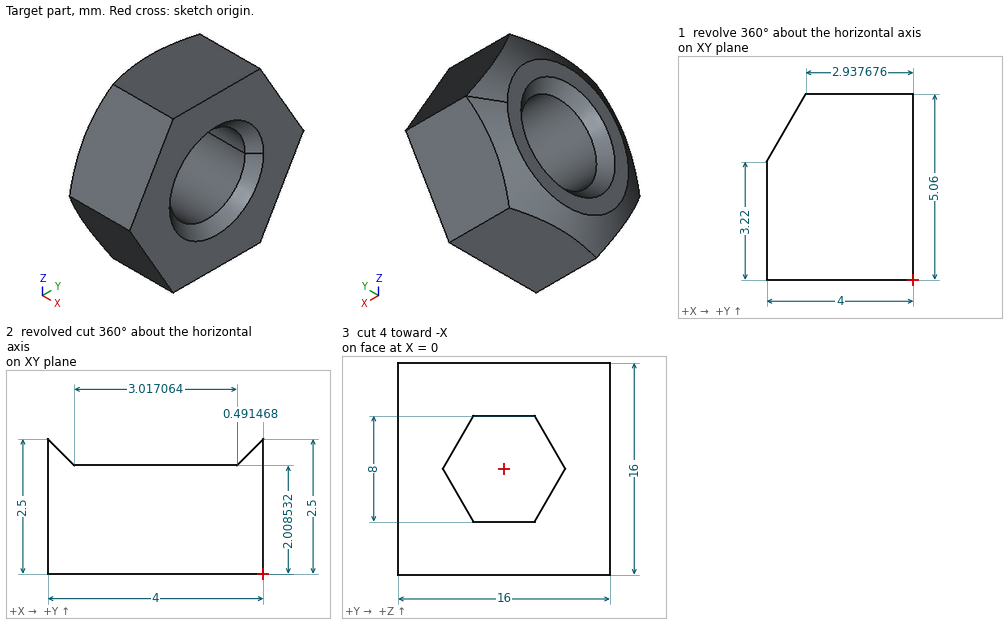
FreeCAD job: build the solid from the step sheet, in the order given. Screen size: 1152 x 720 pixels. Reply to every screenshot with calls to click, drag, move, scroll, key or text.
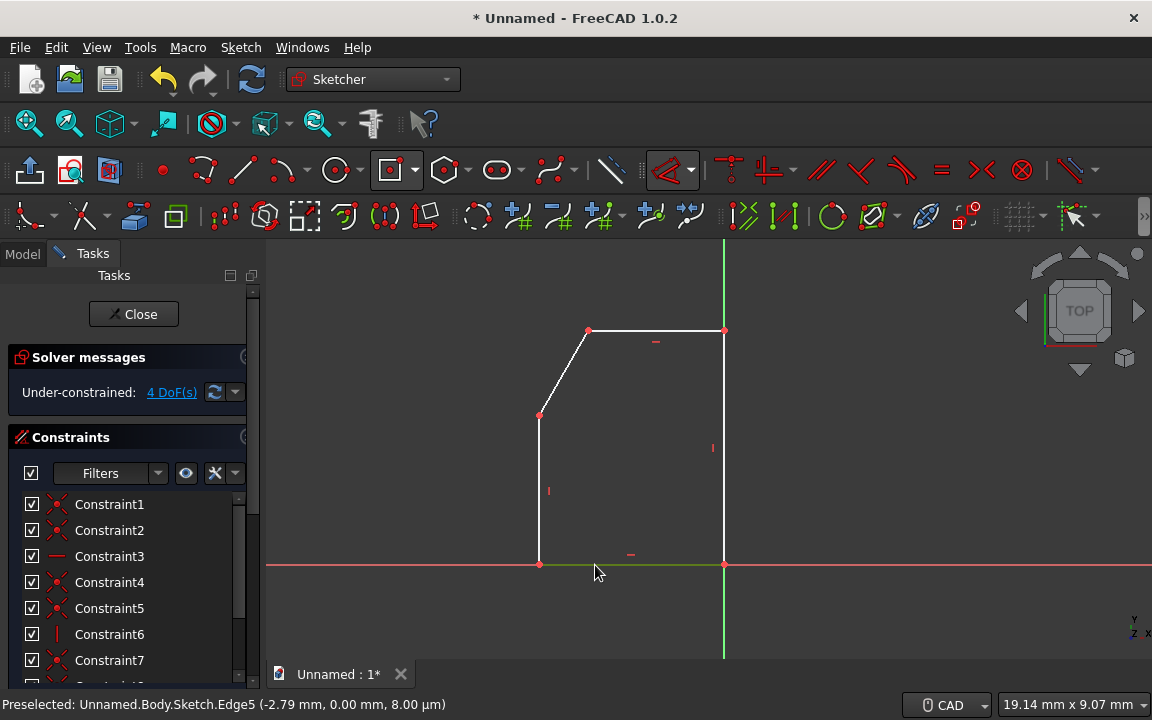
key(l)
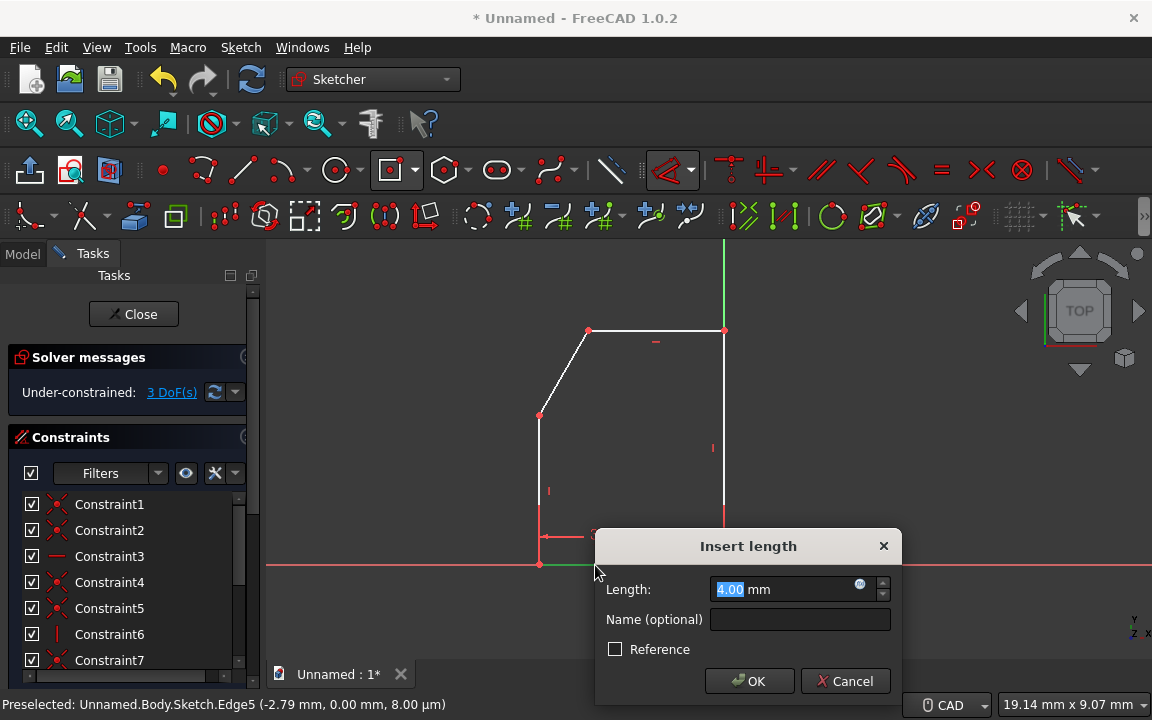
text(4)
key(Return)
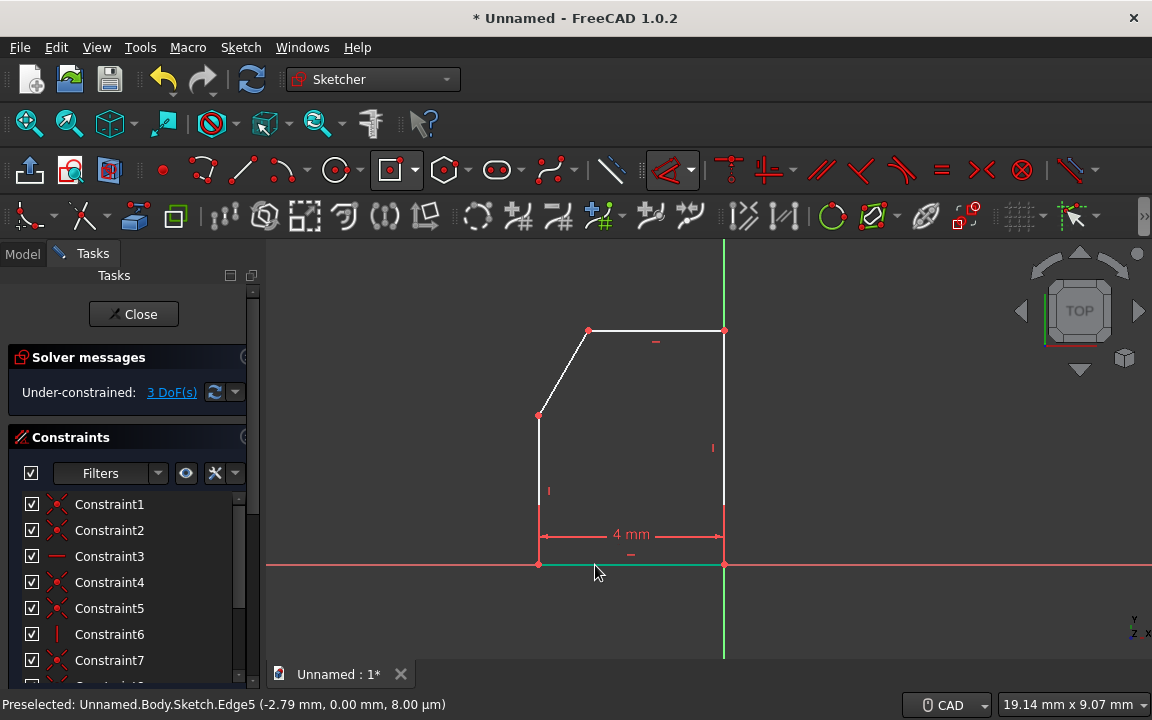
click(724, 494)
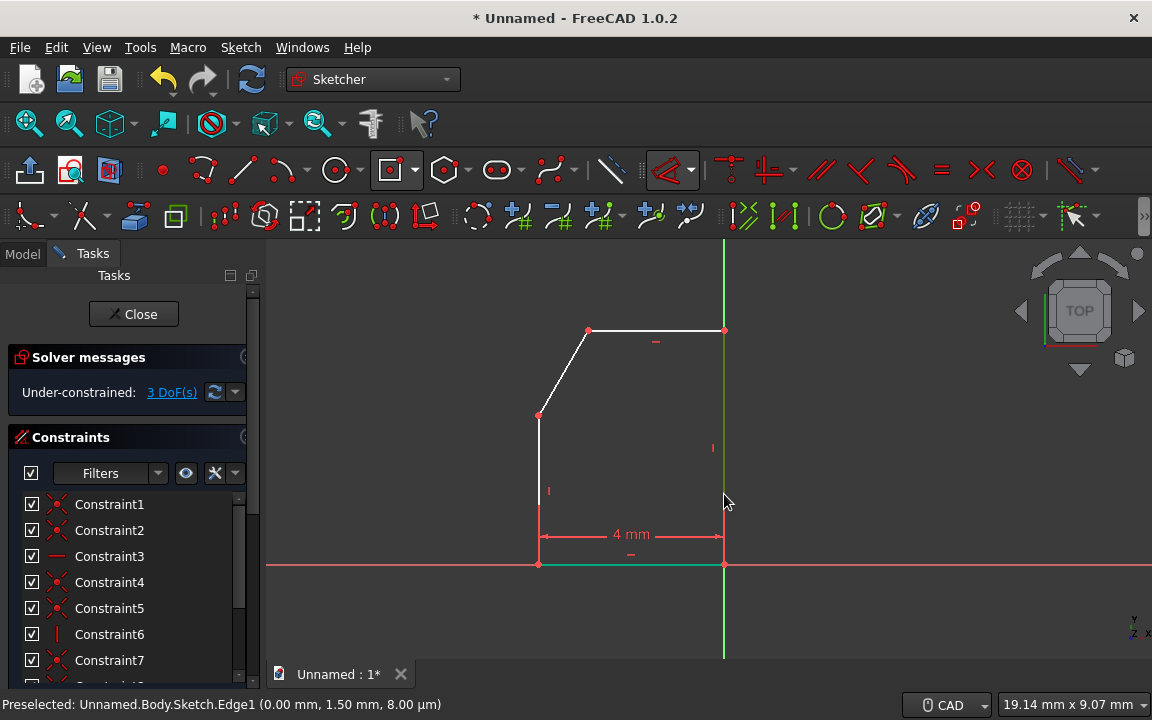
key(i)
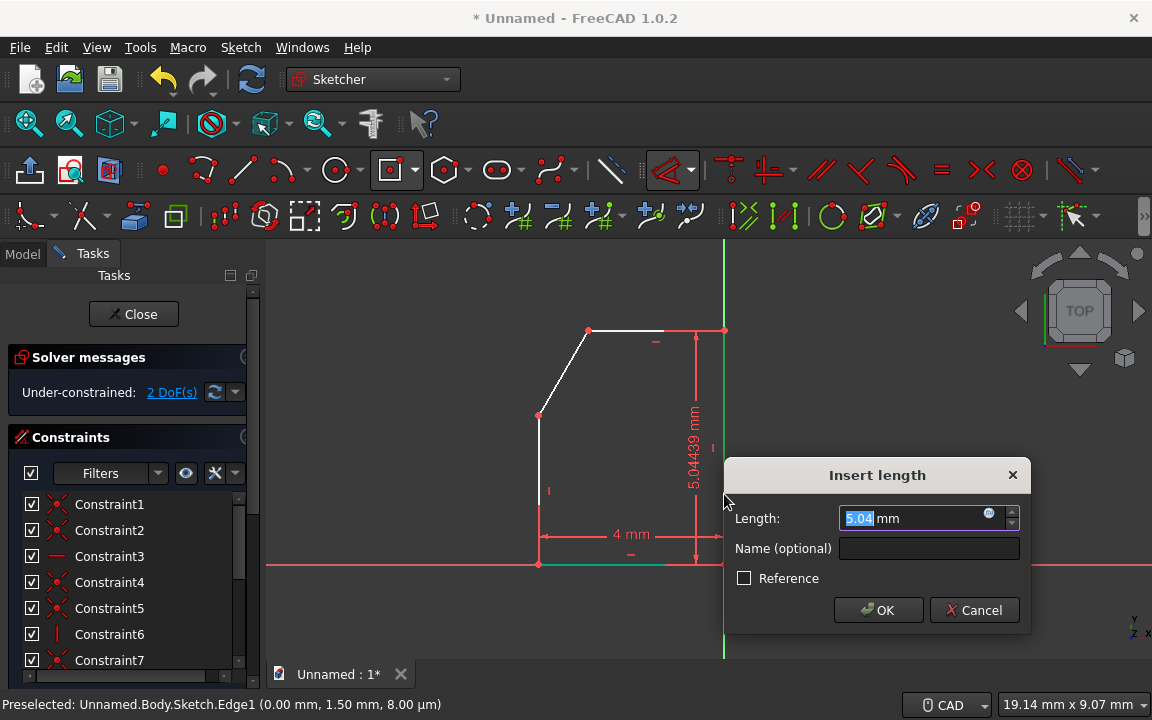
text(5.06)
key(Return)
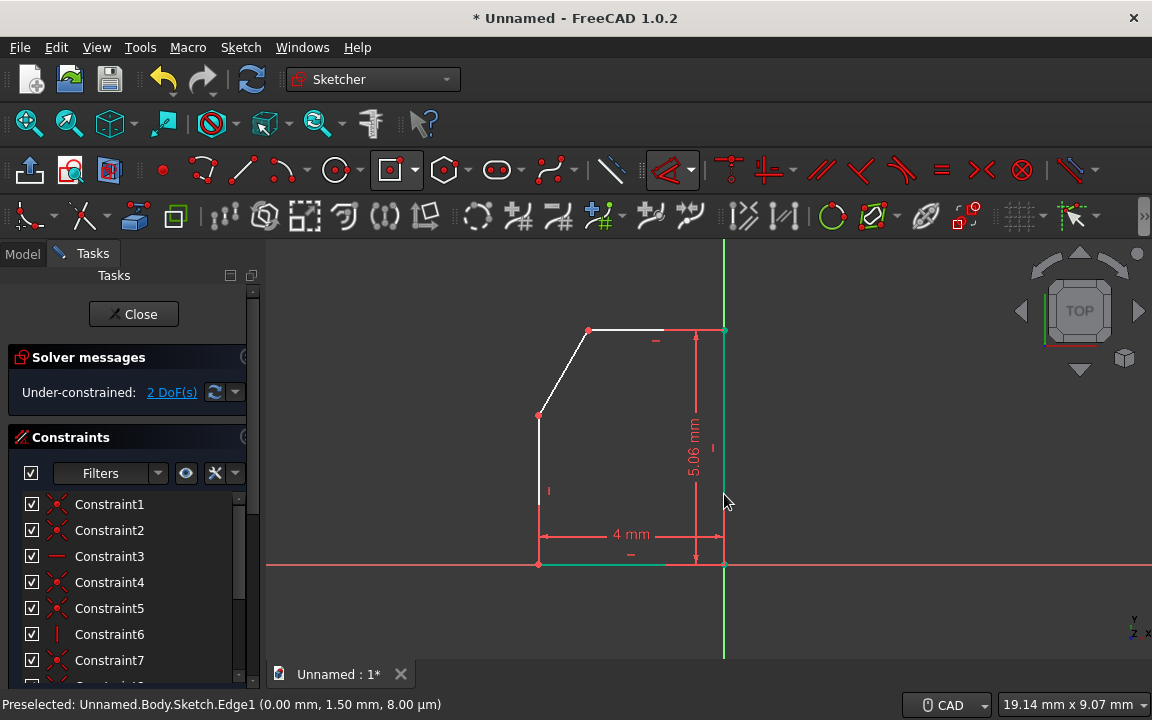
click(539, 461)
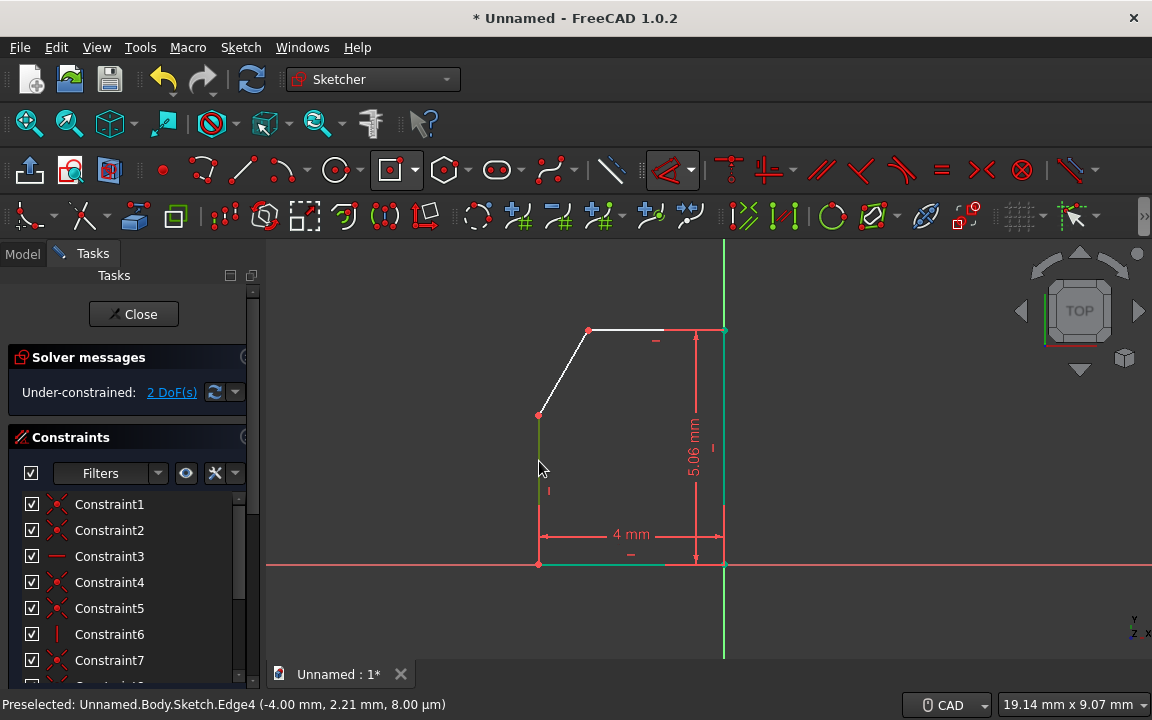
key(i)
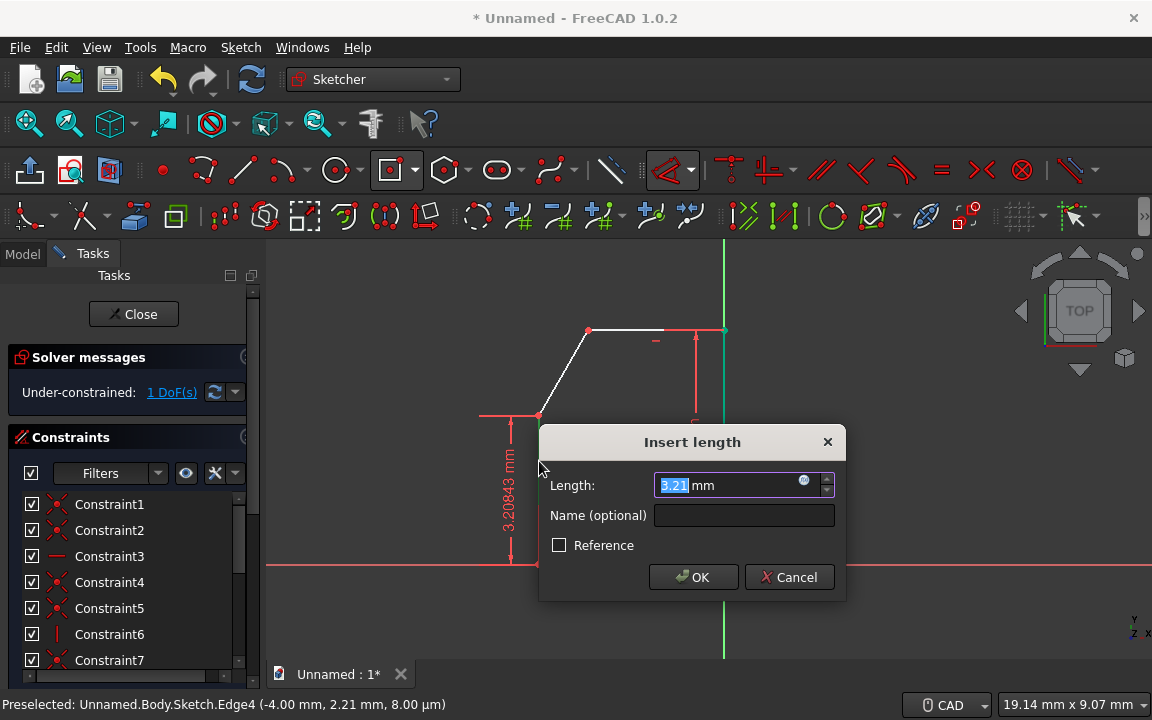
text(3.22)
key(Return)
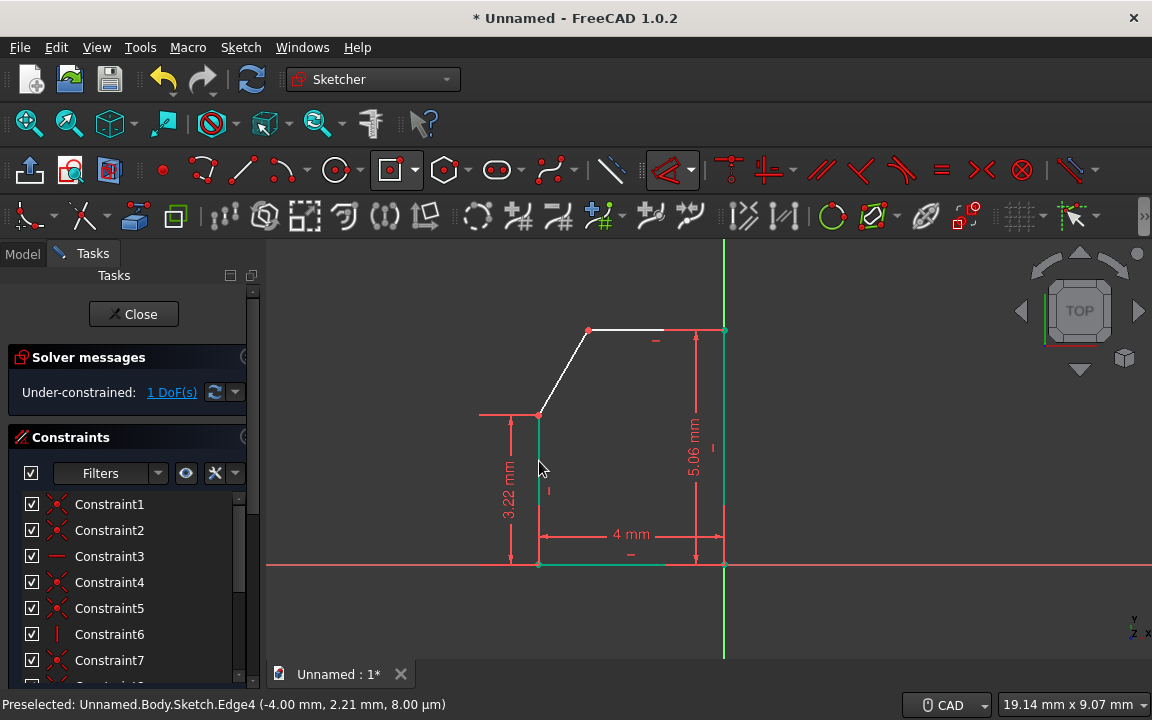
click(683, 330)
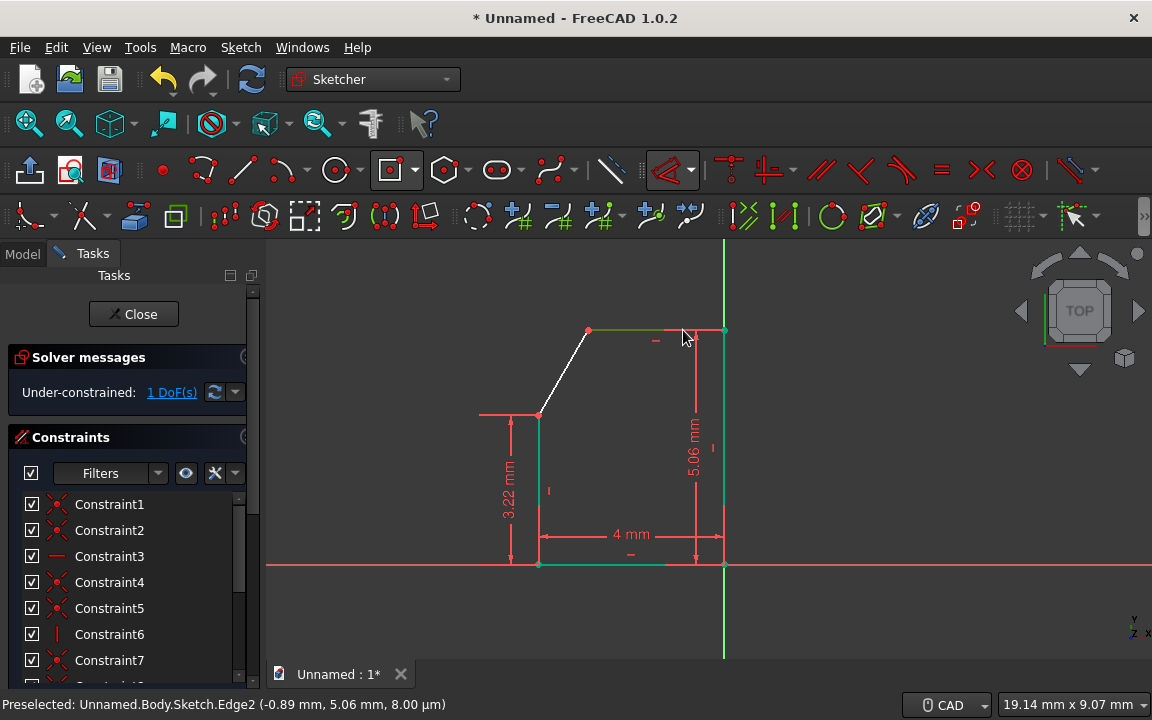
key(l)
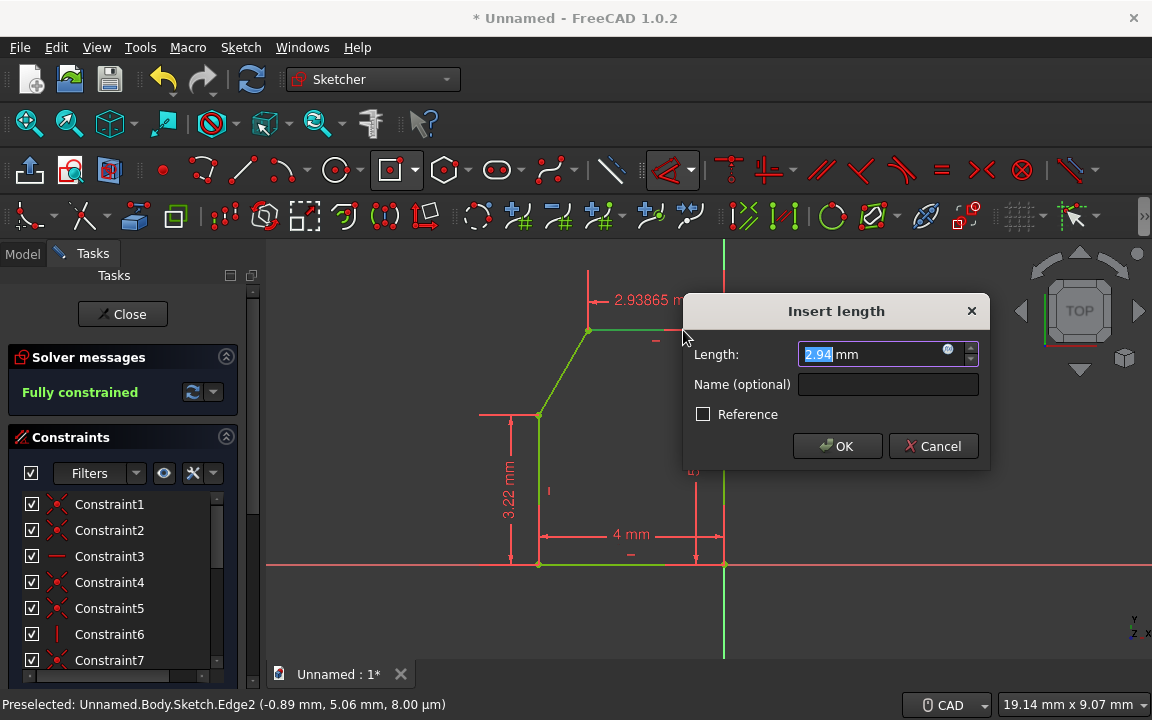
text(2.937676)
key(Return)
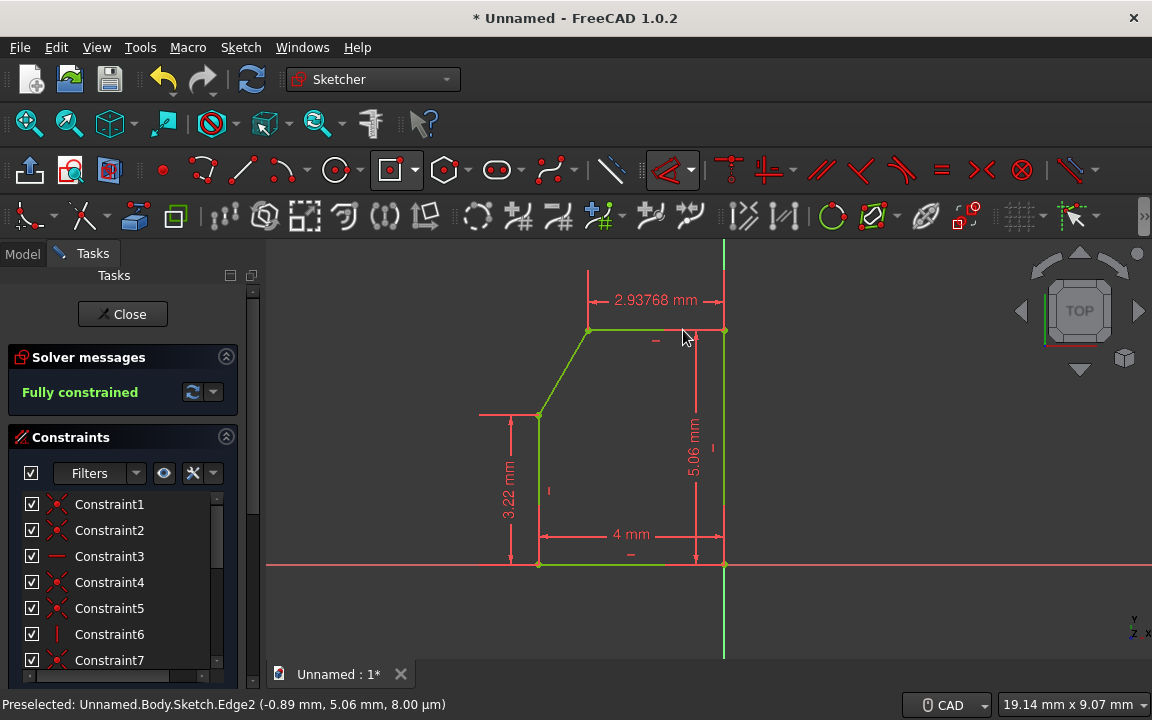
click(123, 314)